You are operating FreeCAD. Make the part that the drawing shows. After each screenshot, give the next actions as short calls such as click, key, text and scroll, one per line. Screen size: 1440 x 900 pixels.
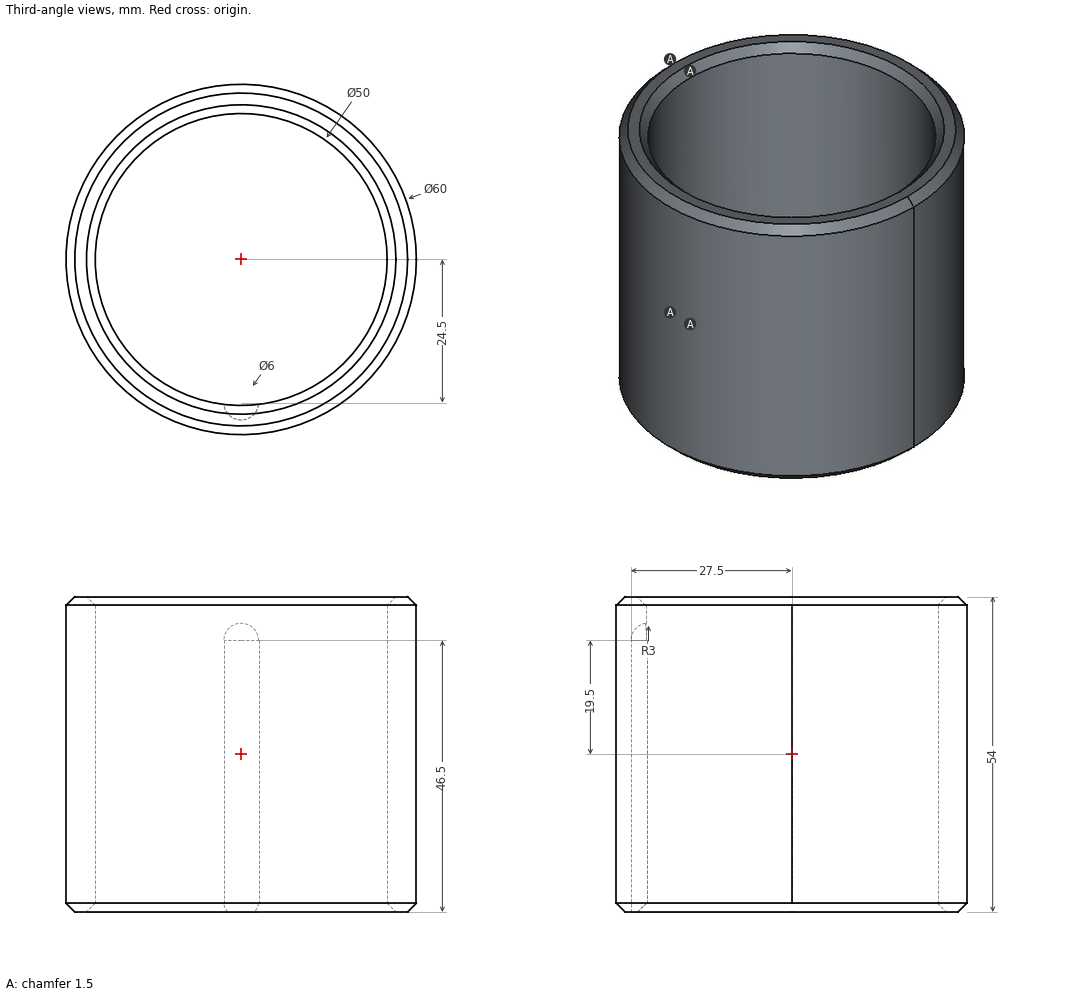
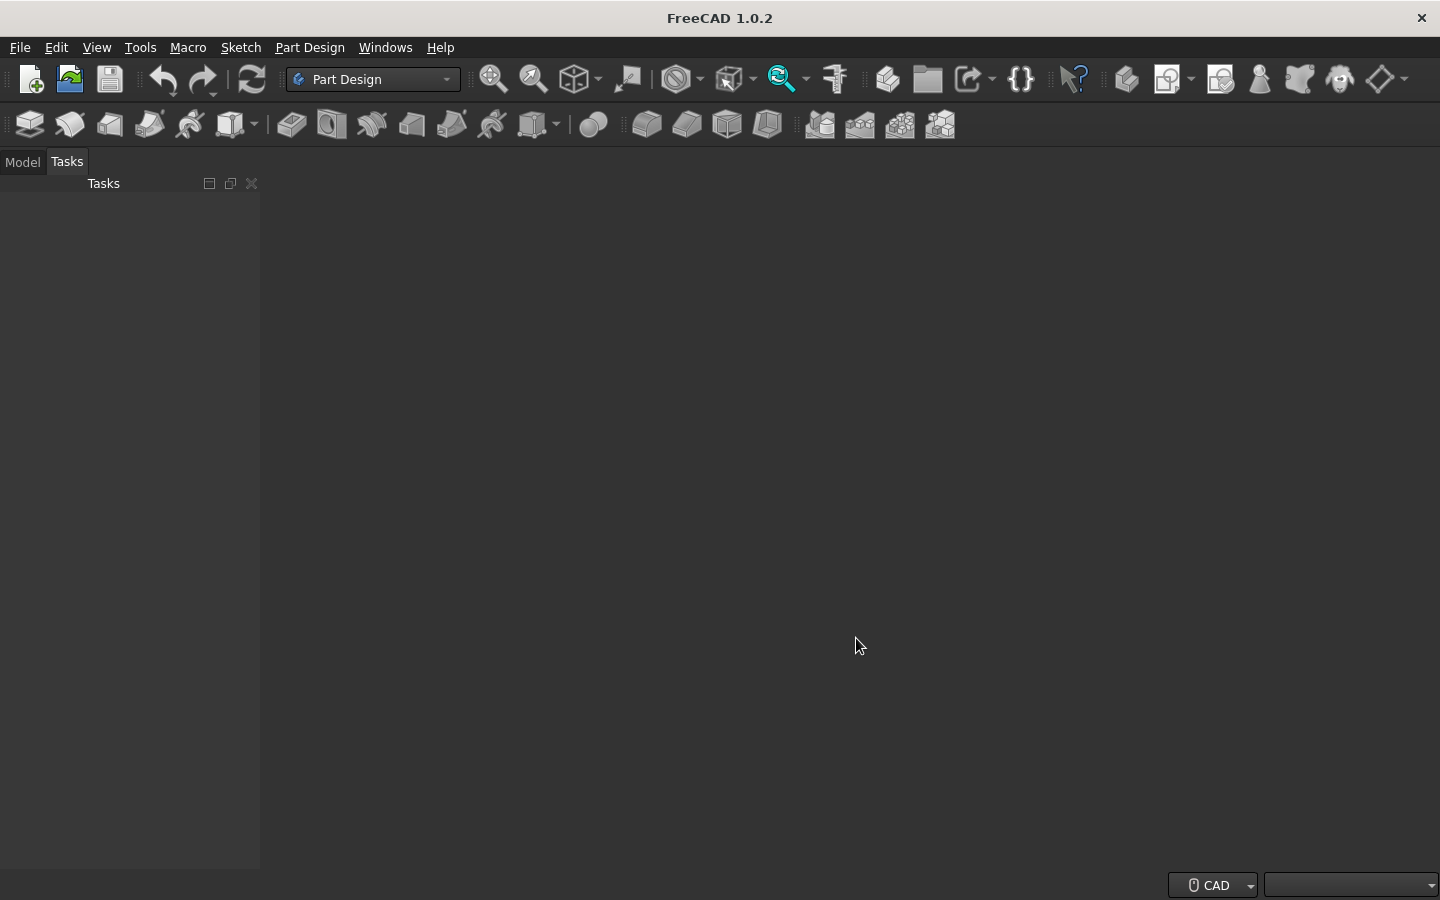
click(30, 80)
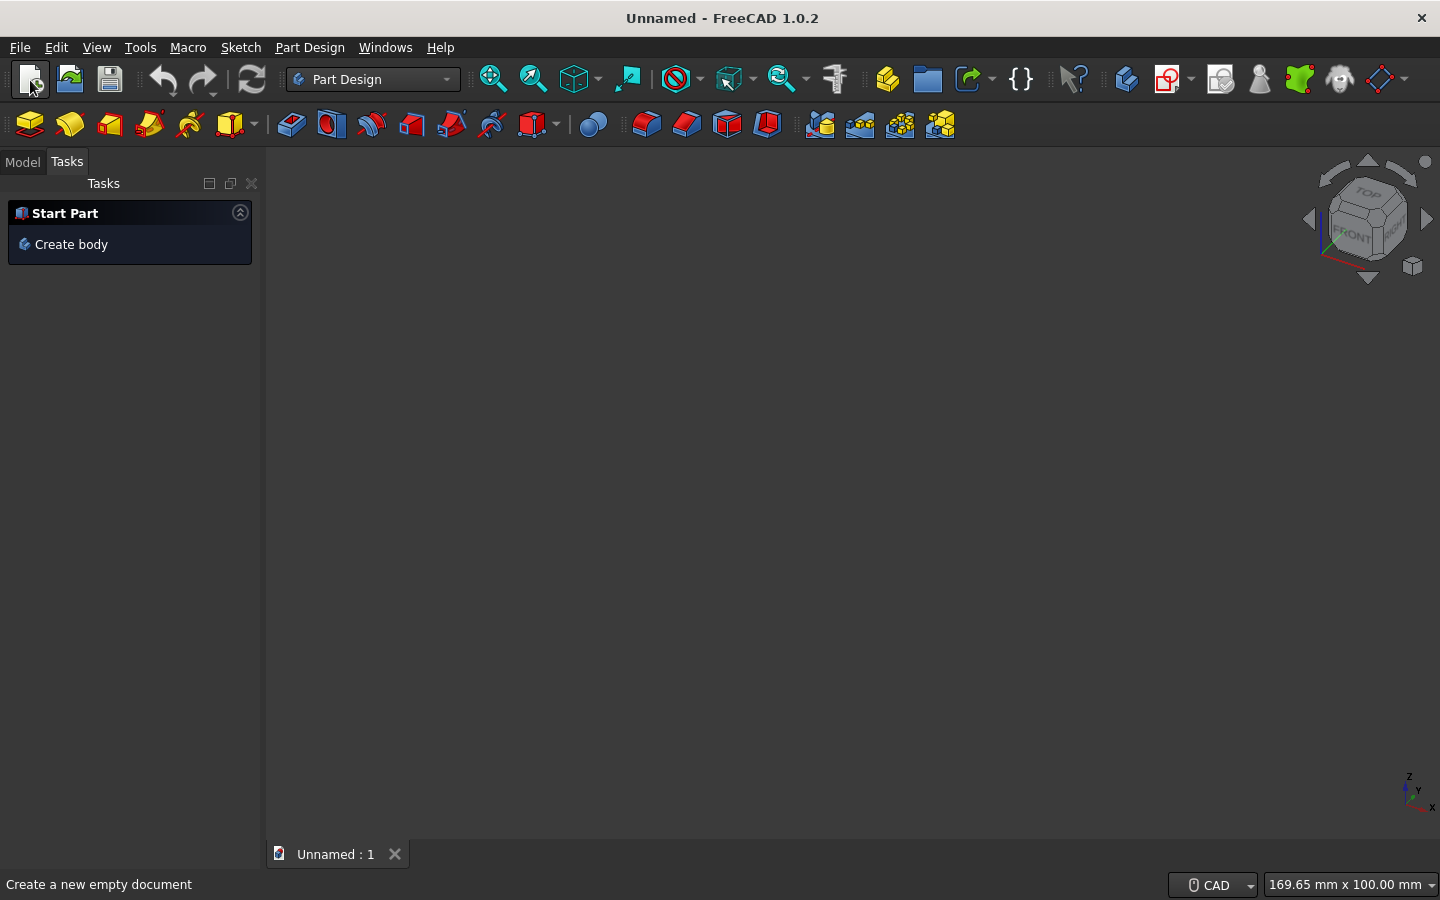
click(1168, 80)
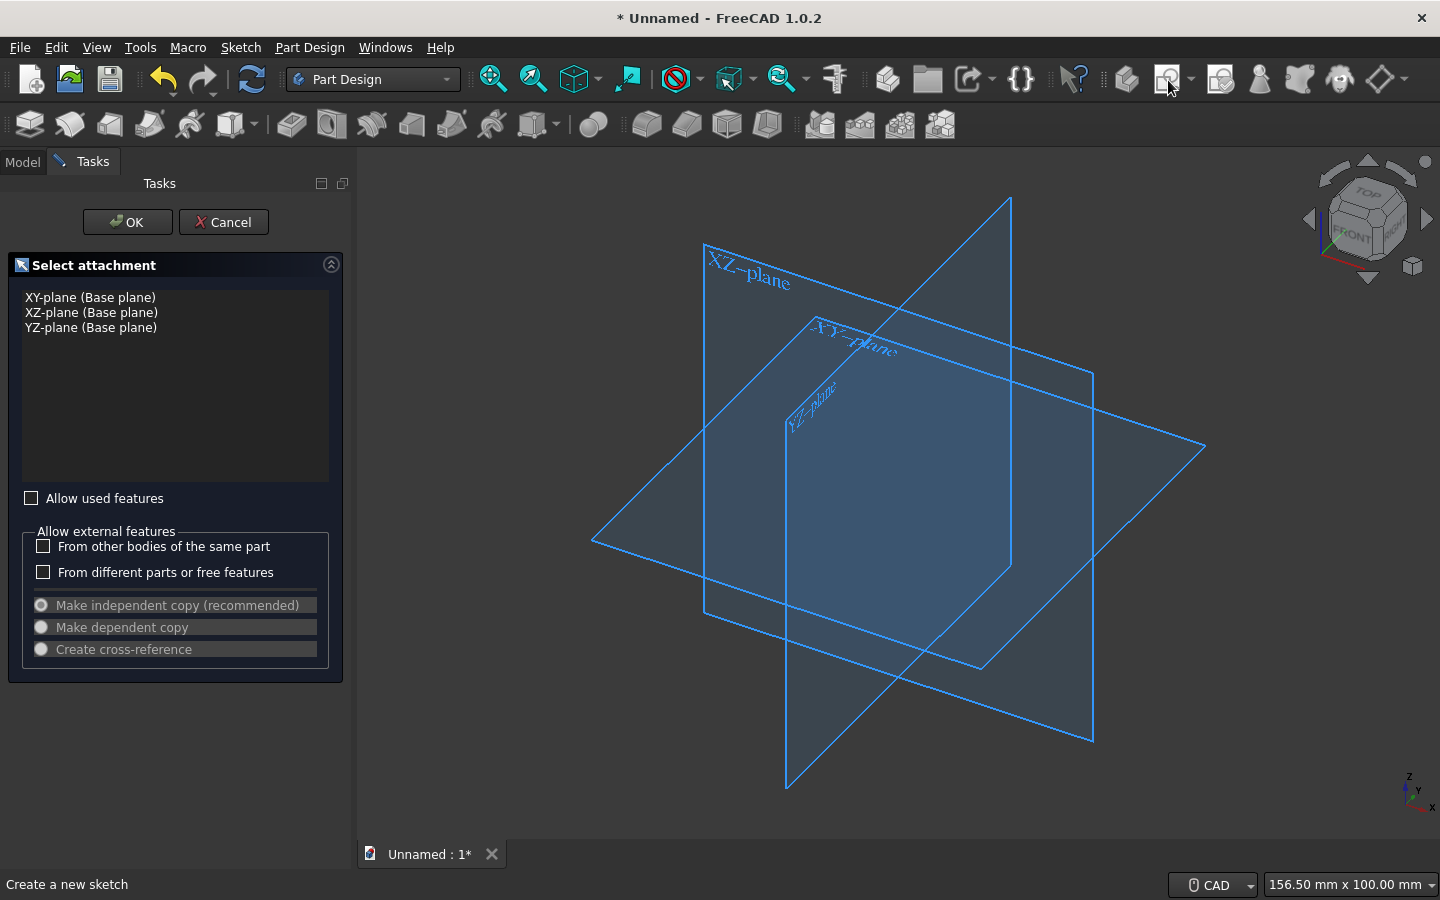
click(82, 298)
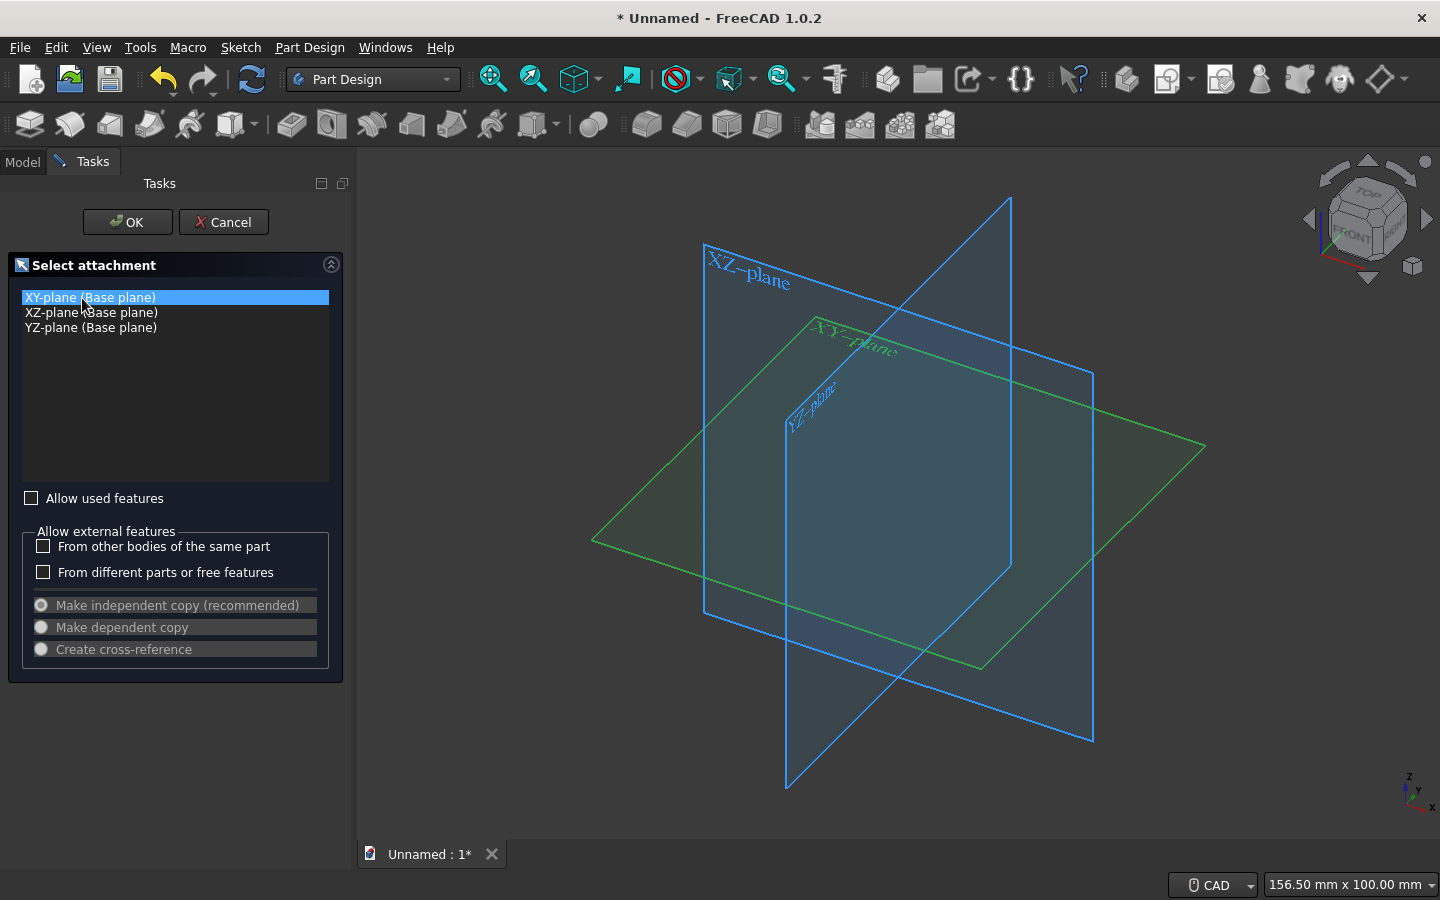
click(128, 222)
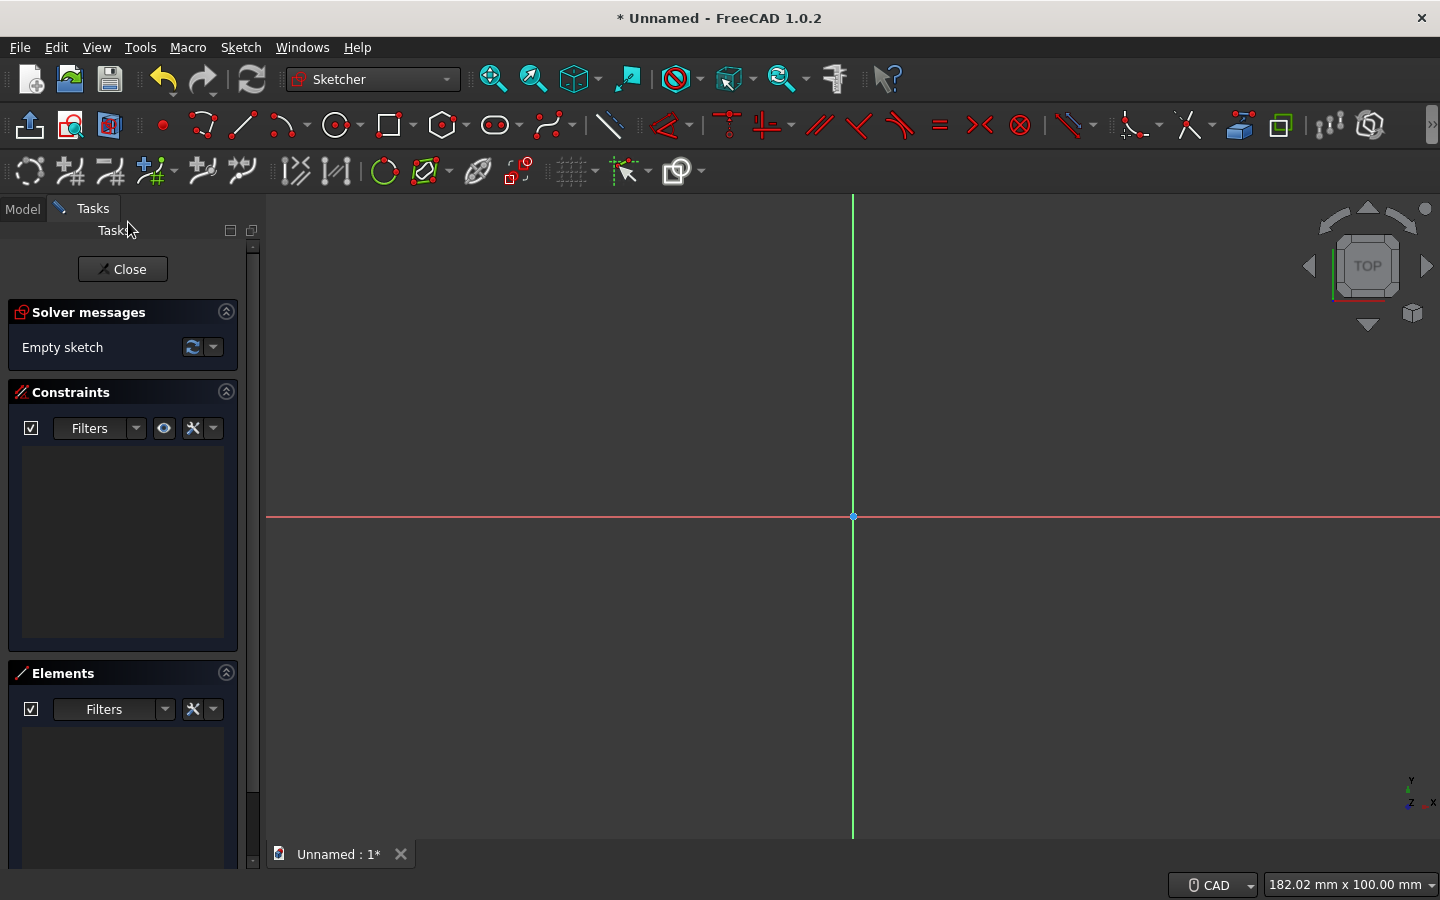
click(336, 126)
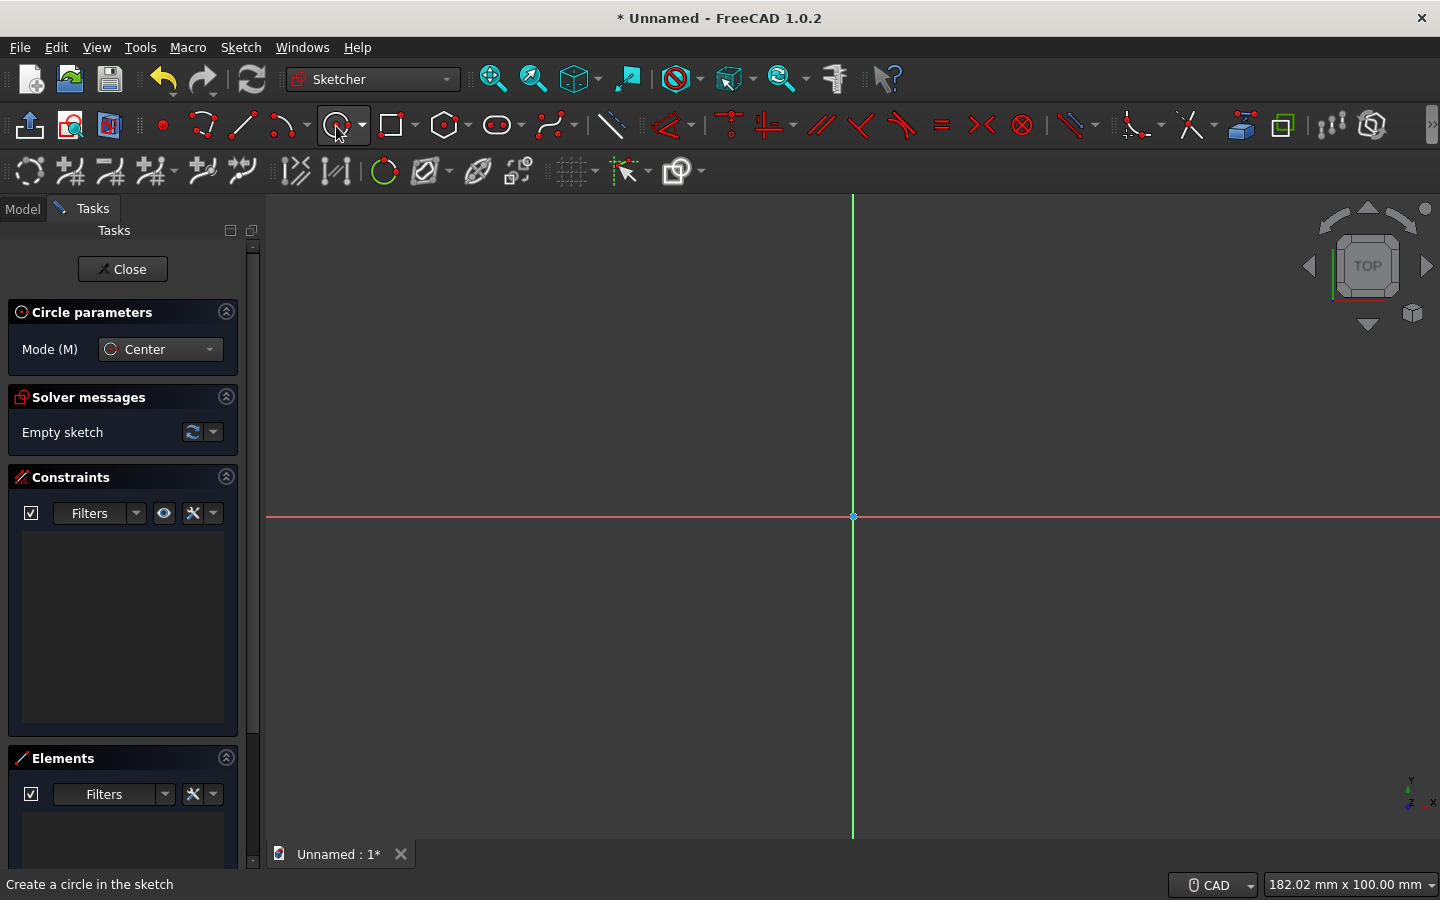
click(853, 516)
click(990, 380)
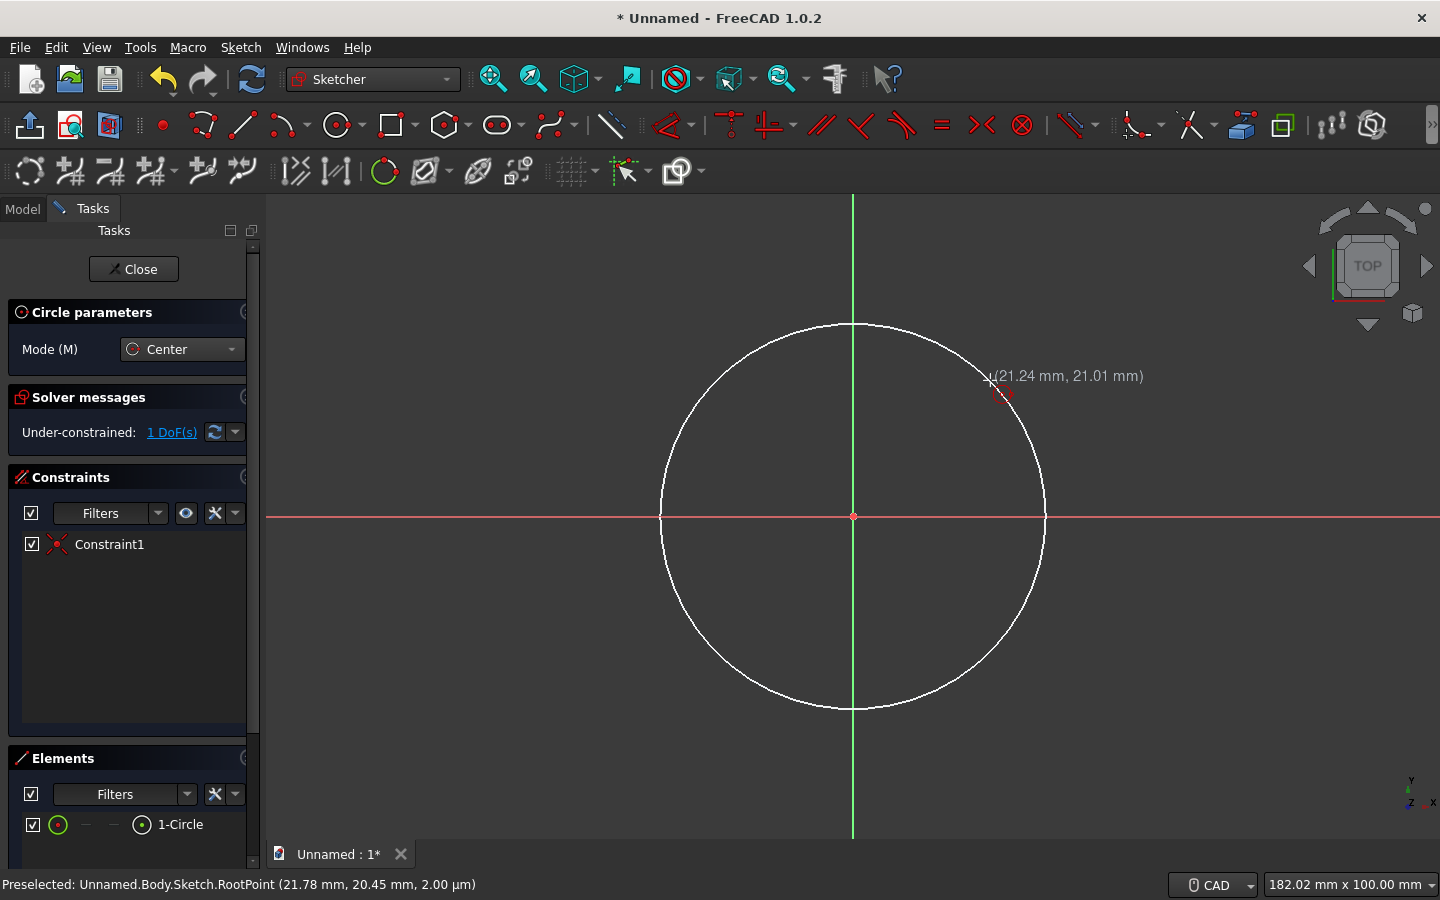
click(853, 516)
click(967, 402)
key(Escape)